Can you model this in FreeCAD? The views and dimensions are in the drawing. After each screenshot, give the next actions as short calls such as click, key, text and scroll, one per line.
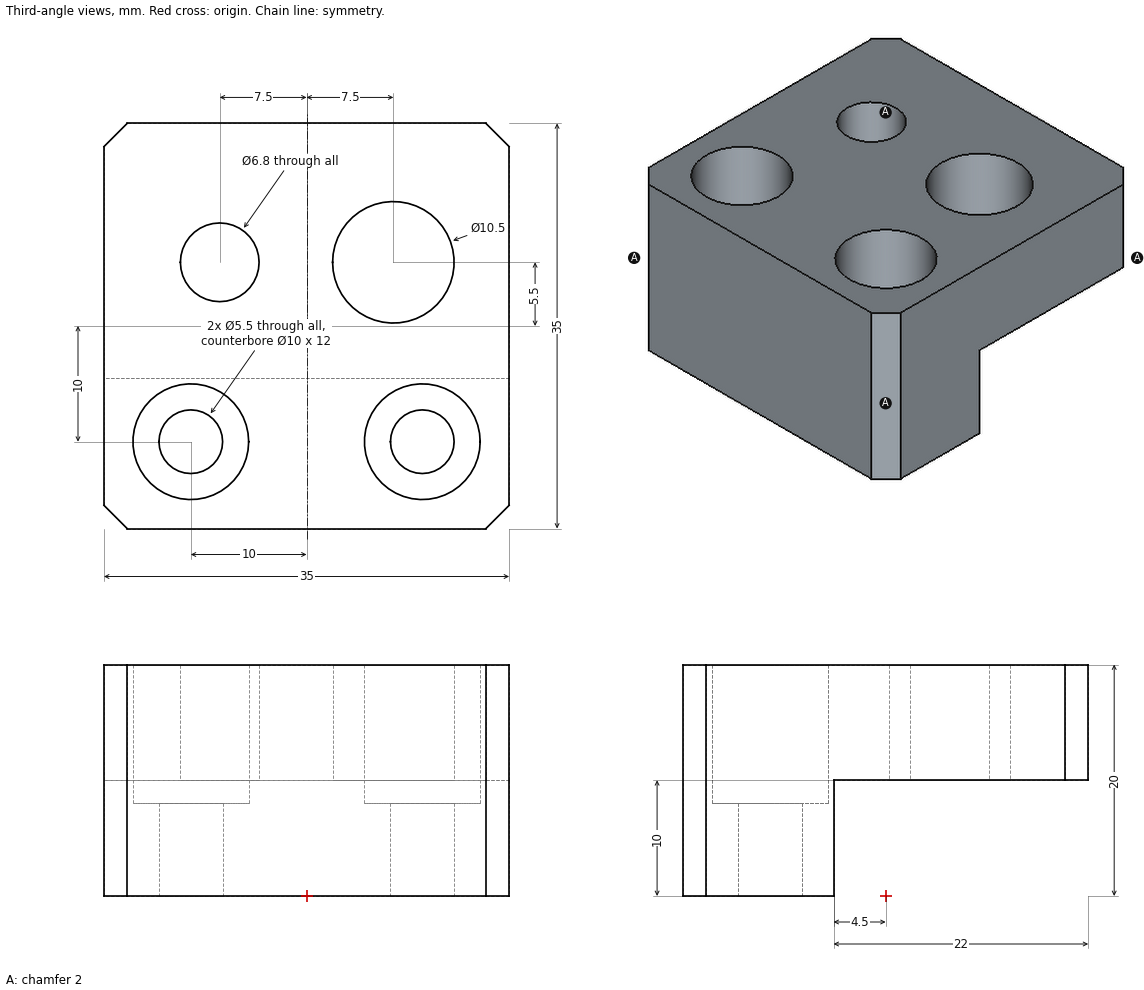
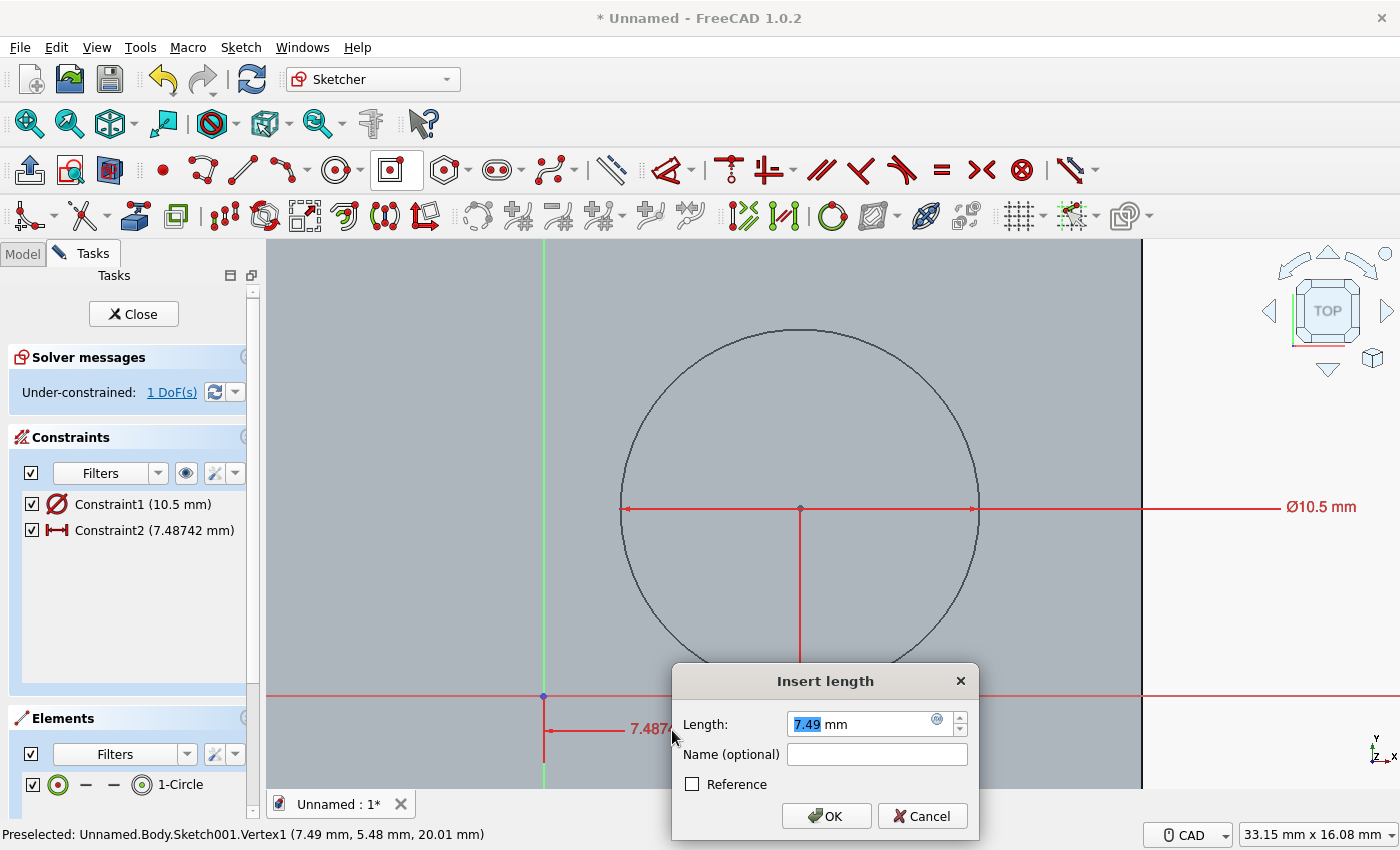
text(7.5)
key(Return)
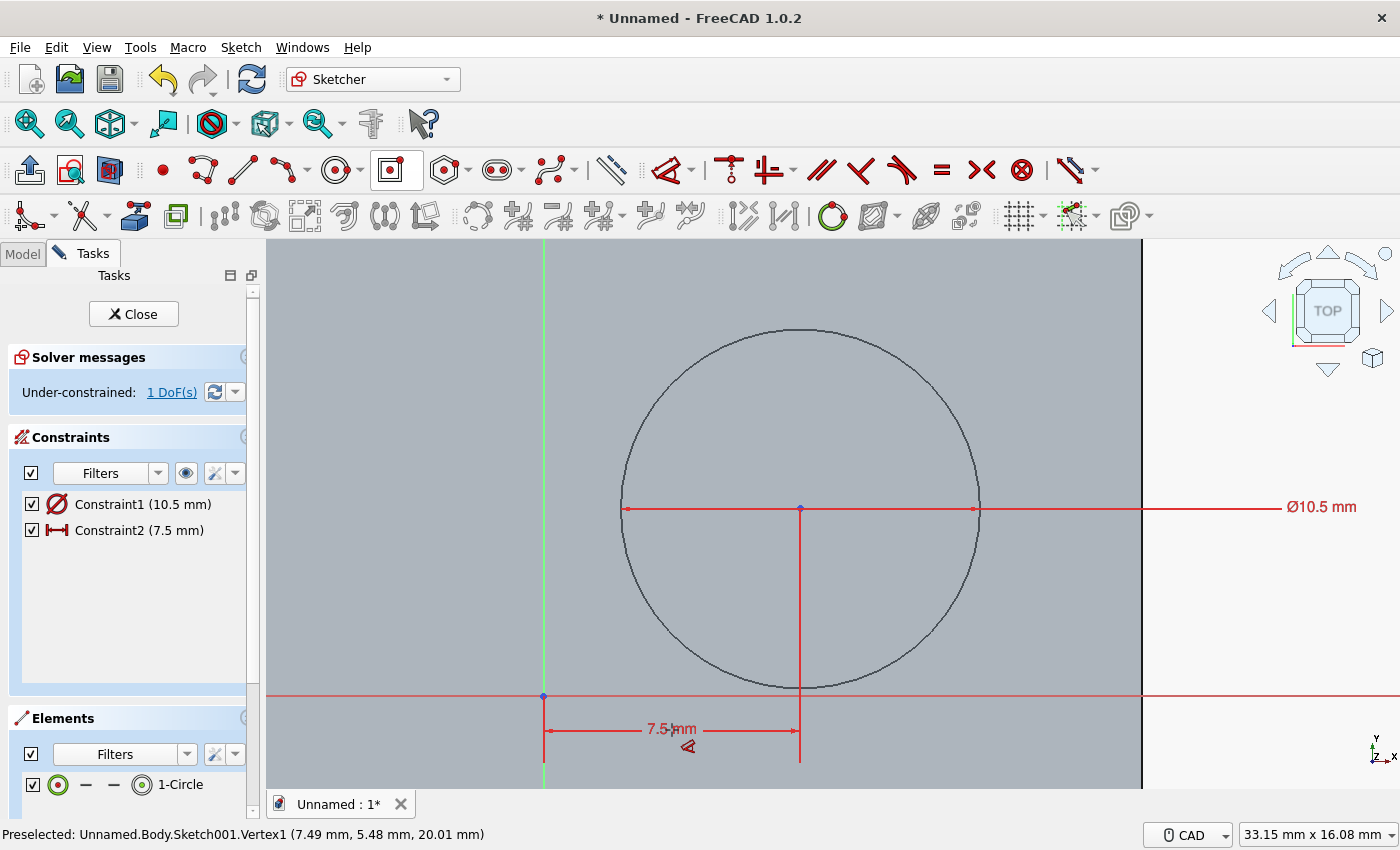
click(800, 509)
click(510, 603)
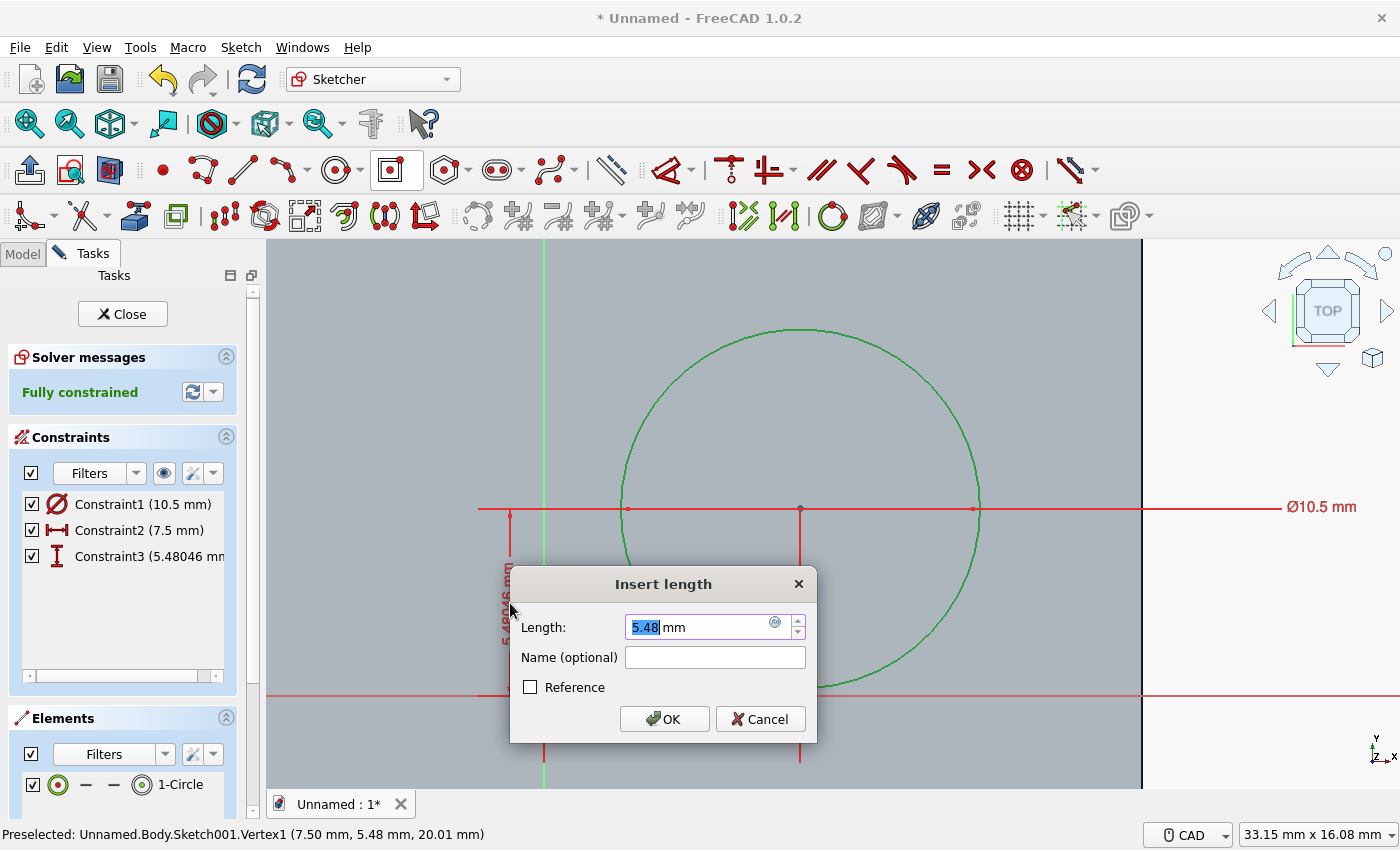
text(5.5)
key(Return)
key(Escape)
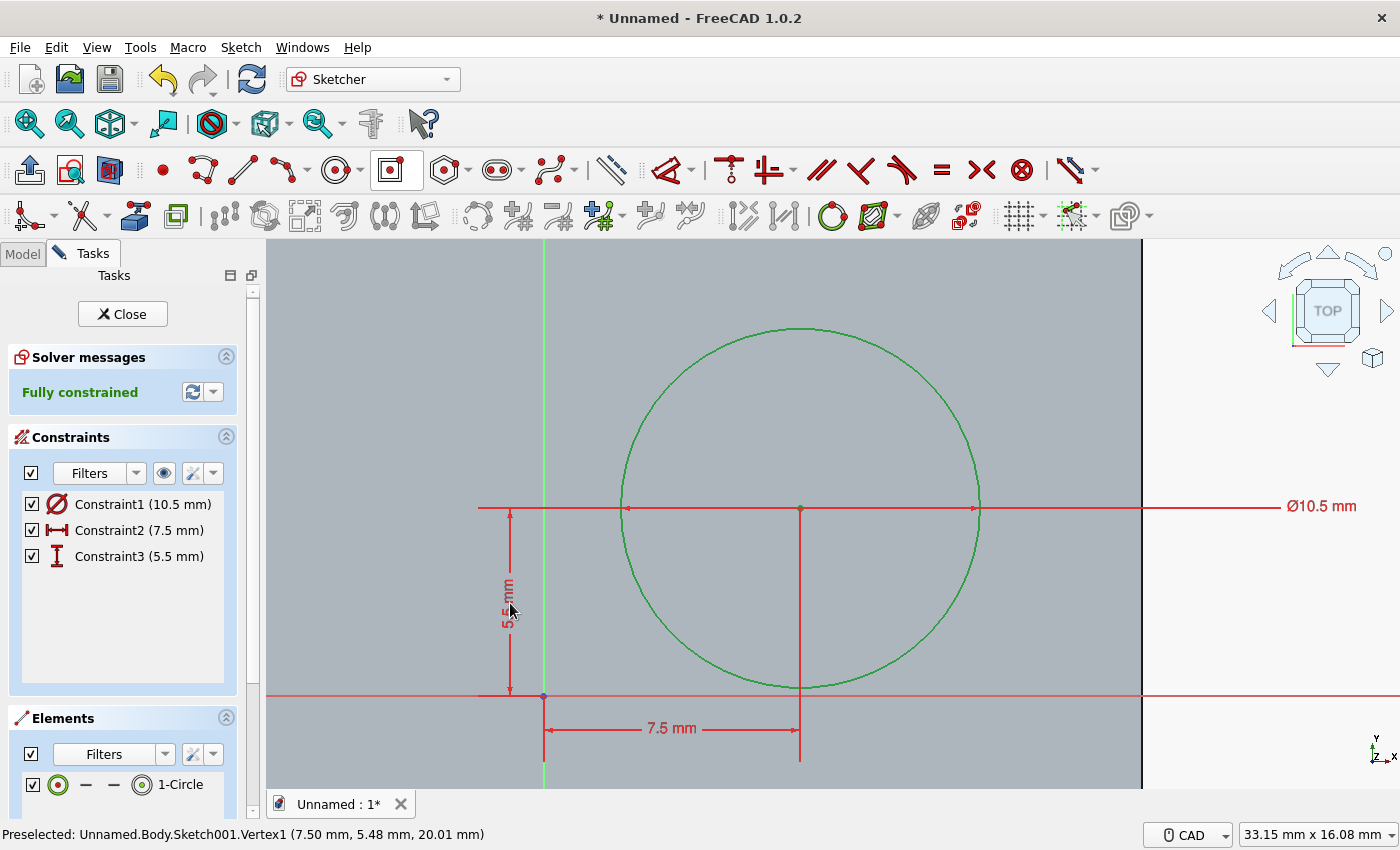
click(123, 314)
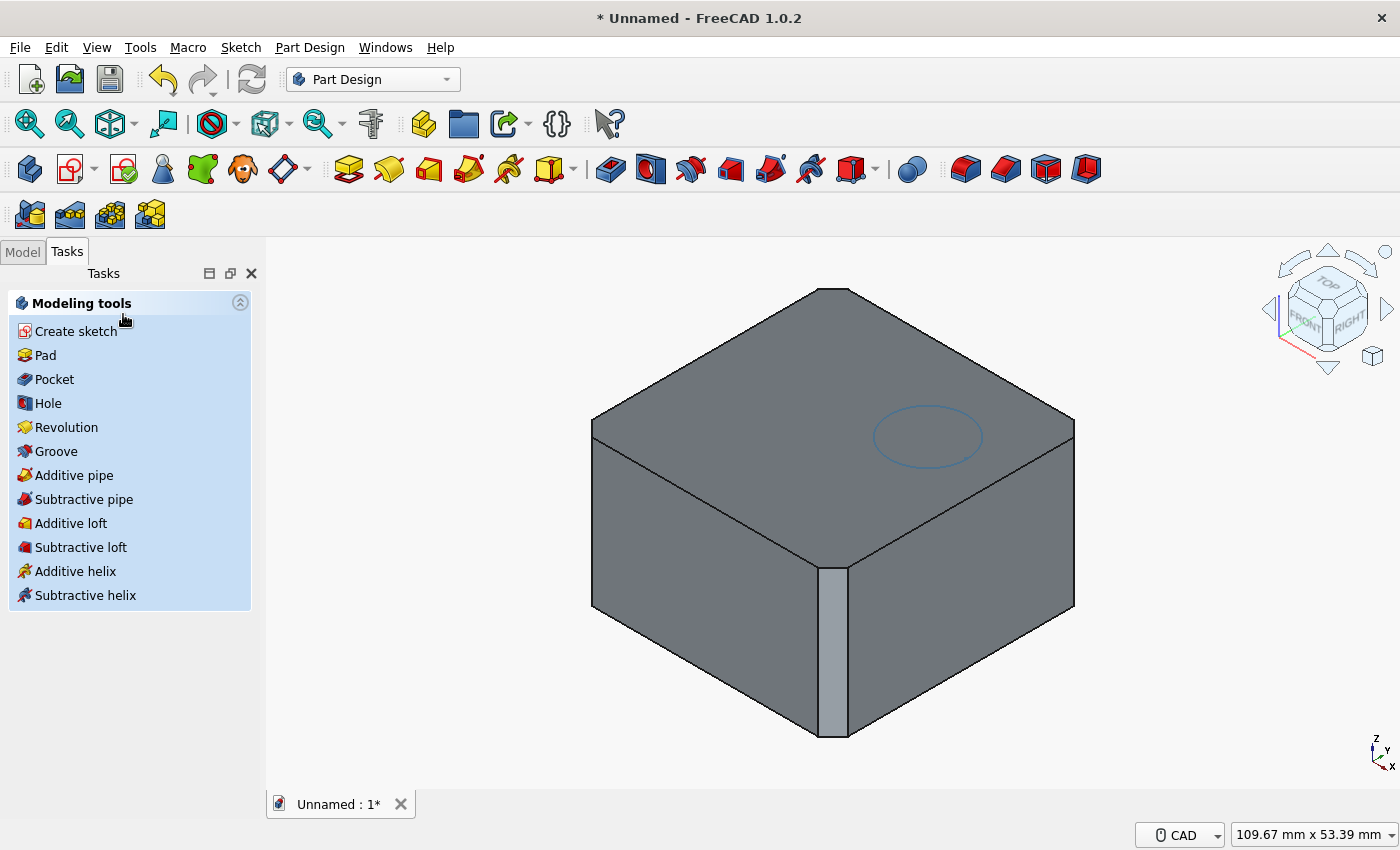
click(612, 170)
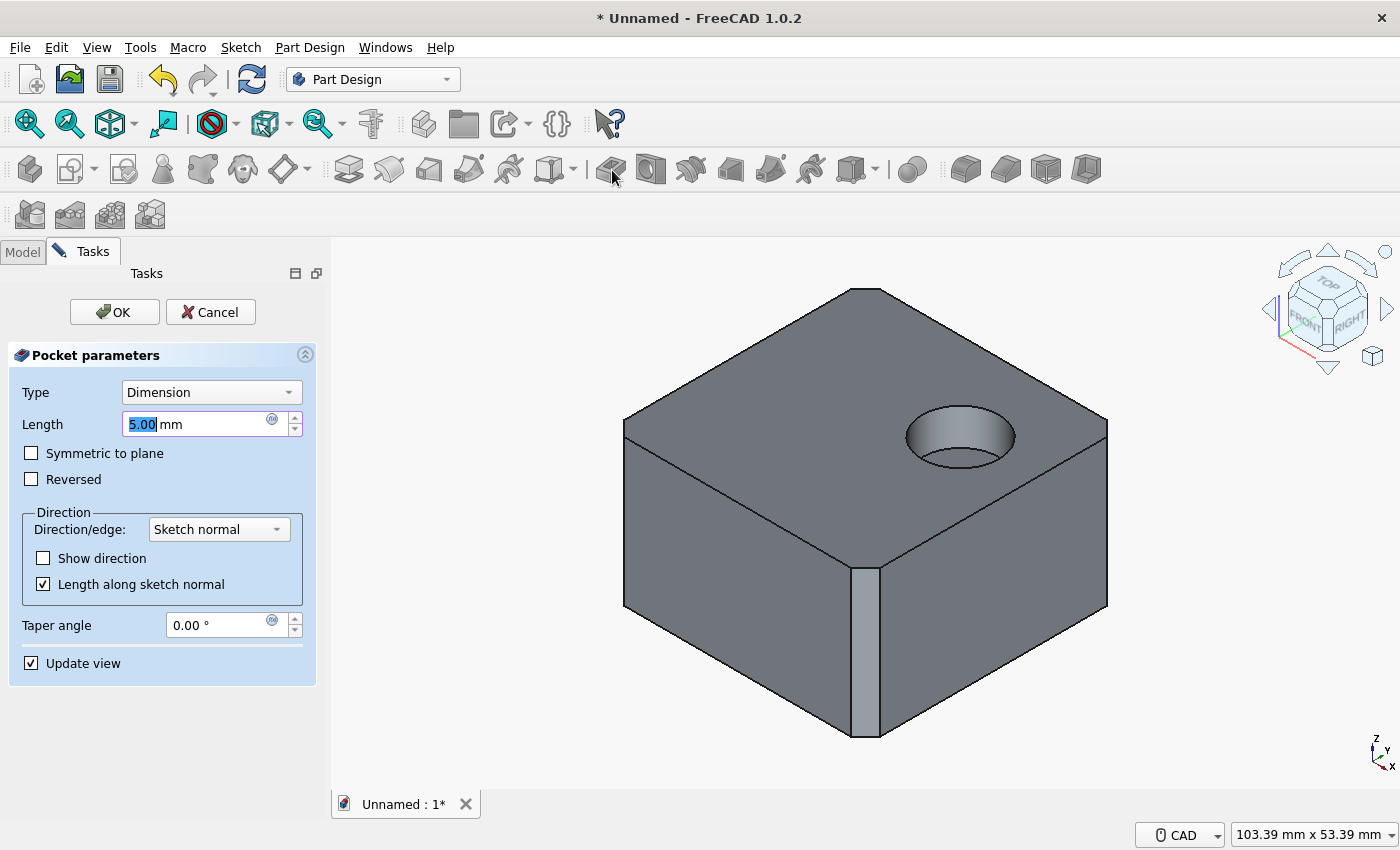
click(212, 392)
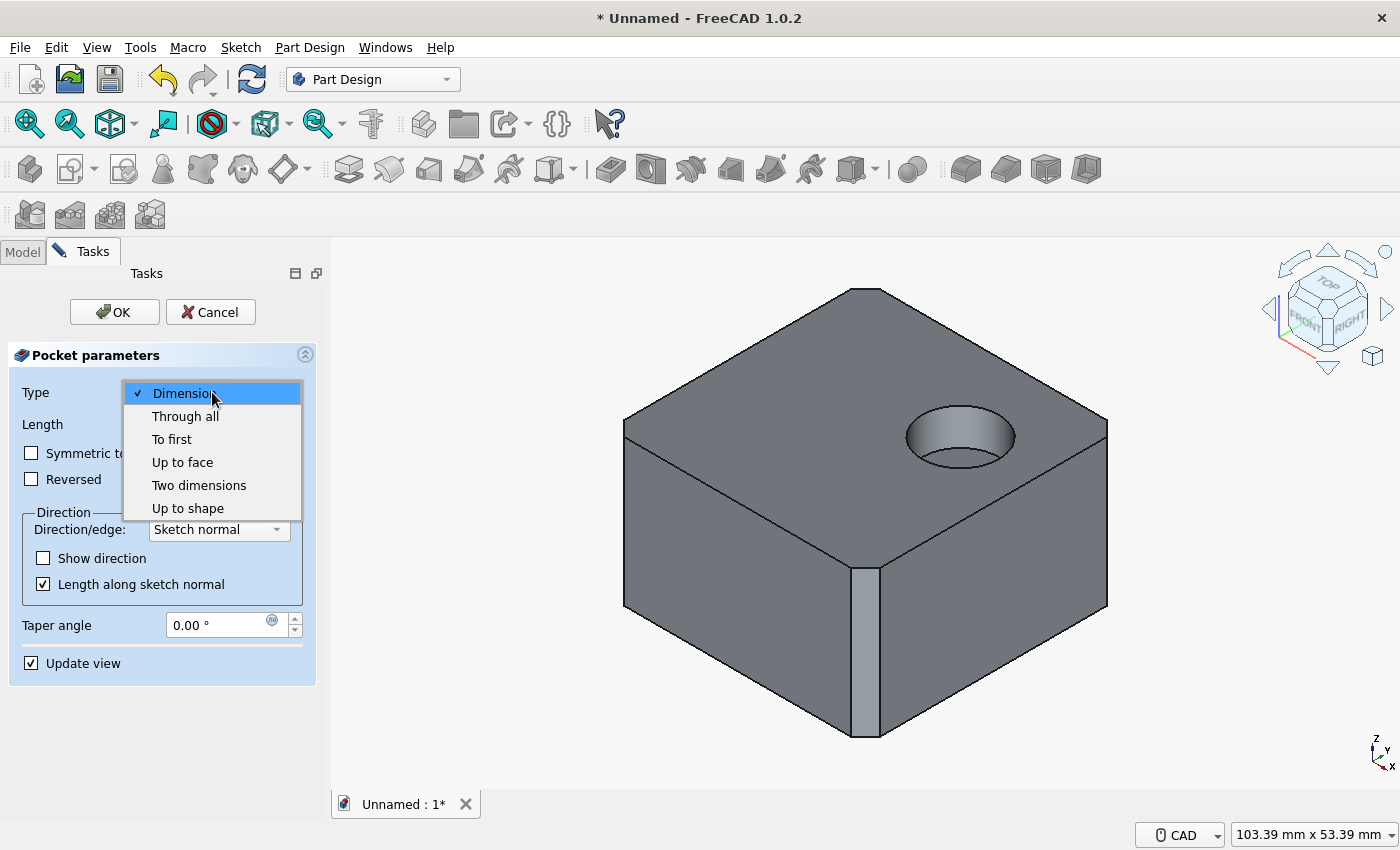
click(212, 416)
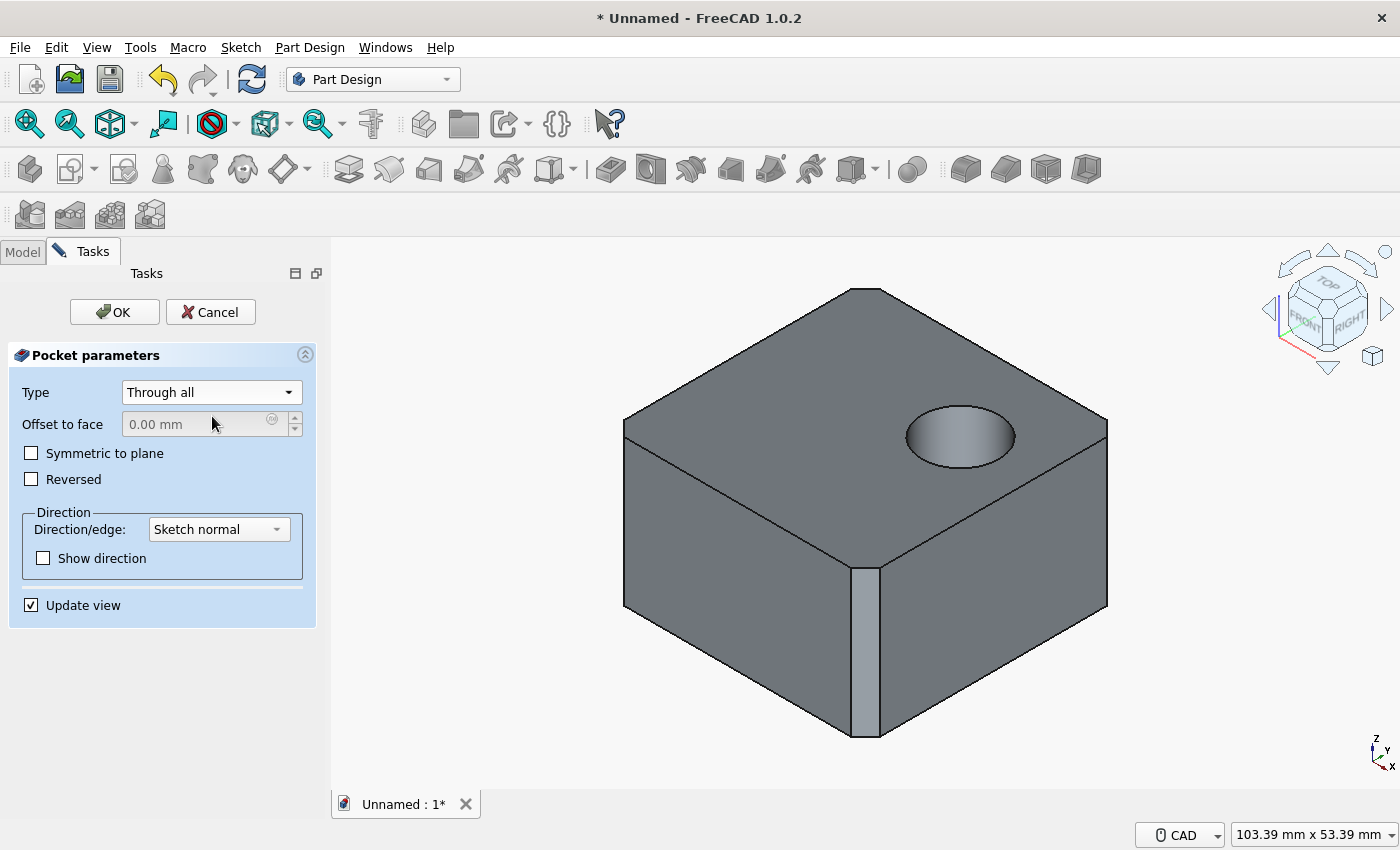
click(115, 312)